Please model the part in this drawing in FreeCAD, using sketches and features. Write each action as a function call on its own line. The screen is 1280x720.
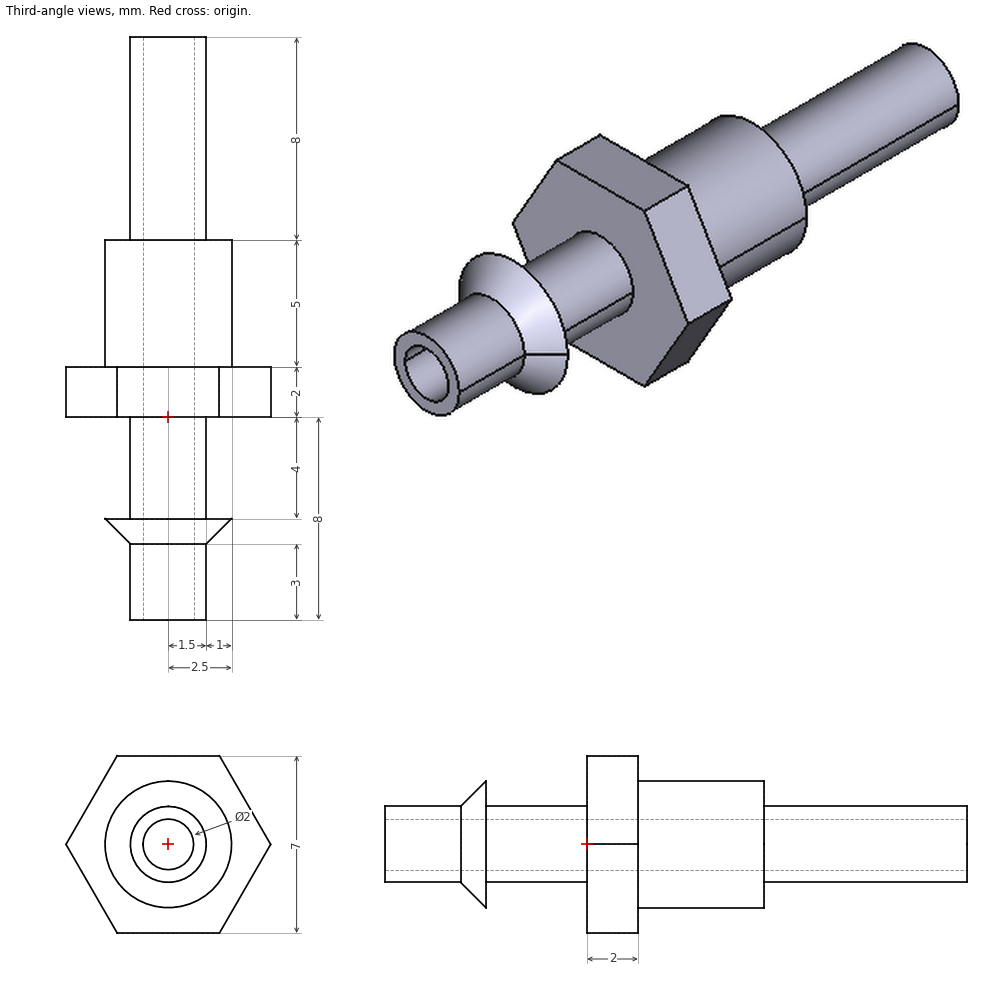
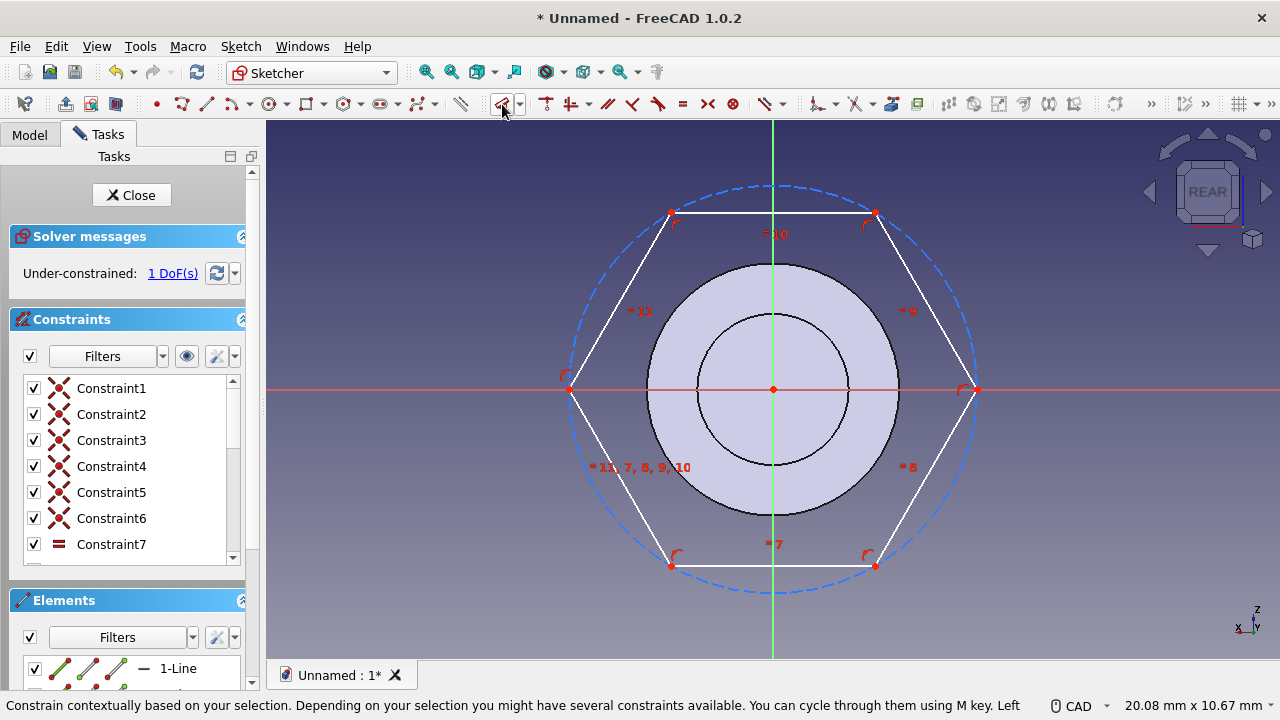
click(671, 566)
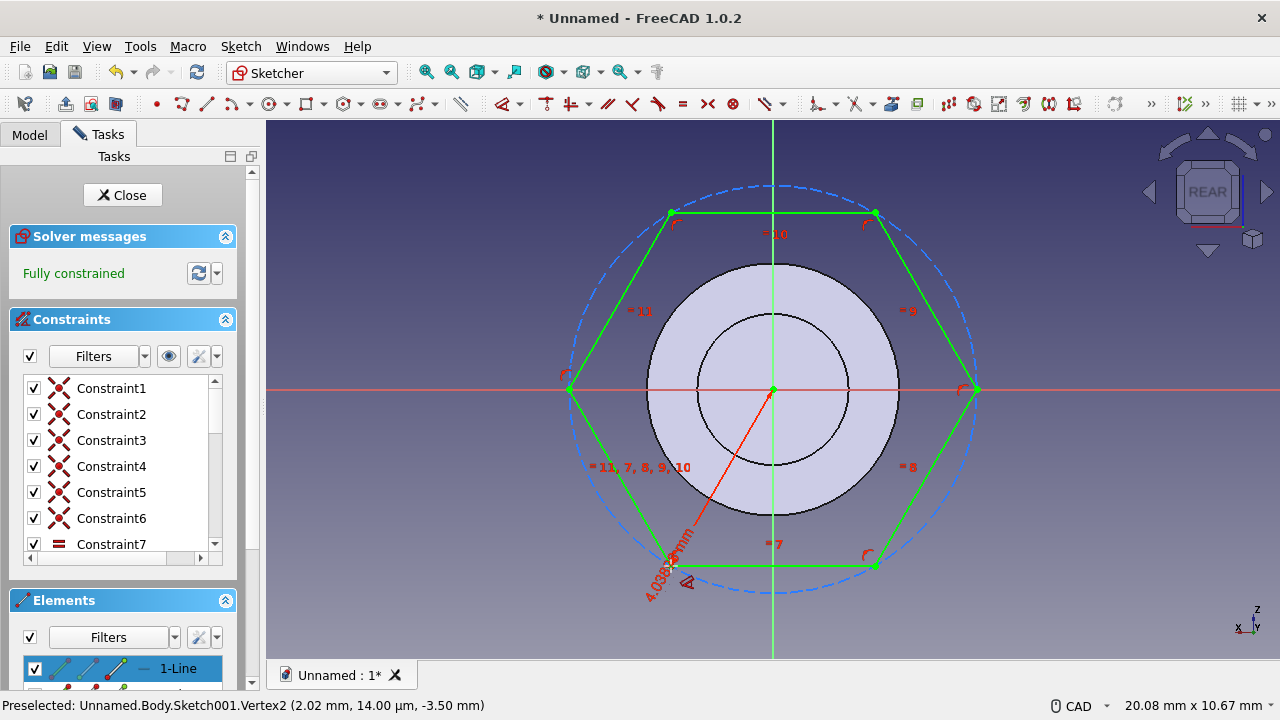
click(875, 213)
click(909, 308)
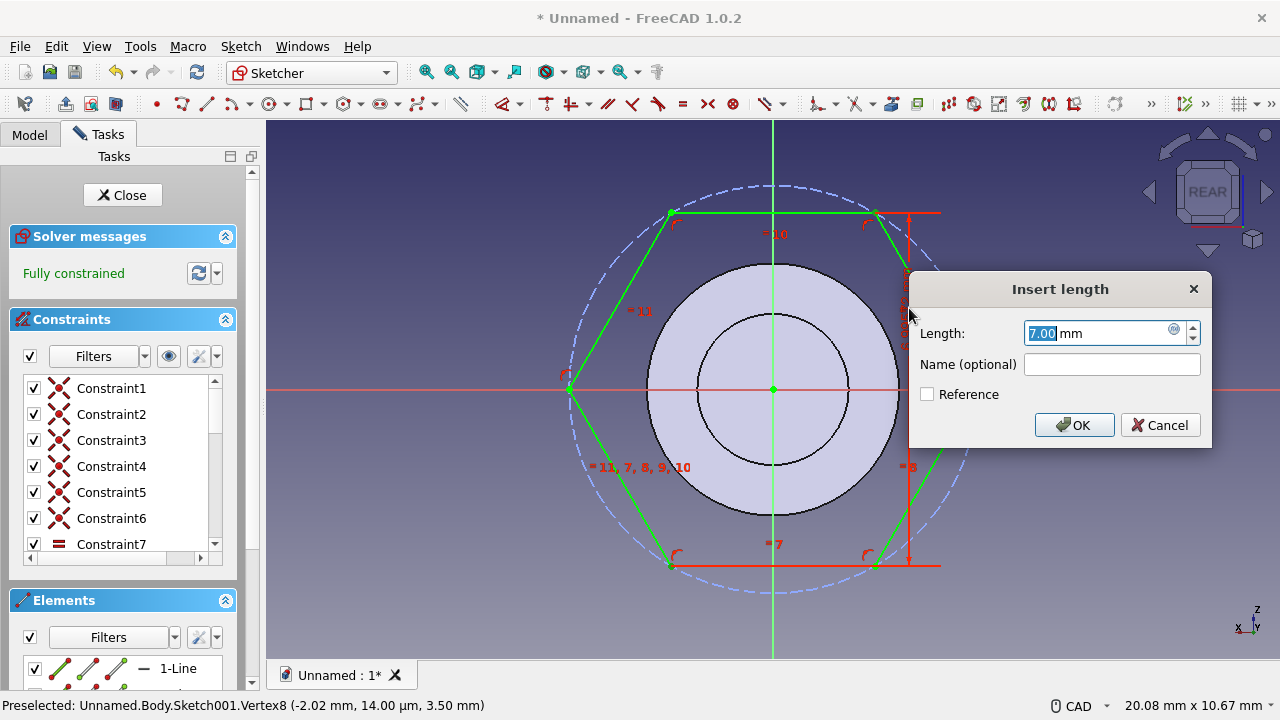
text(7)
key(Return)
key(Escape)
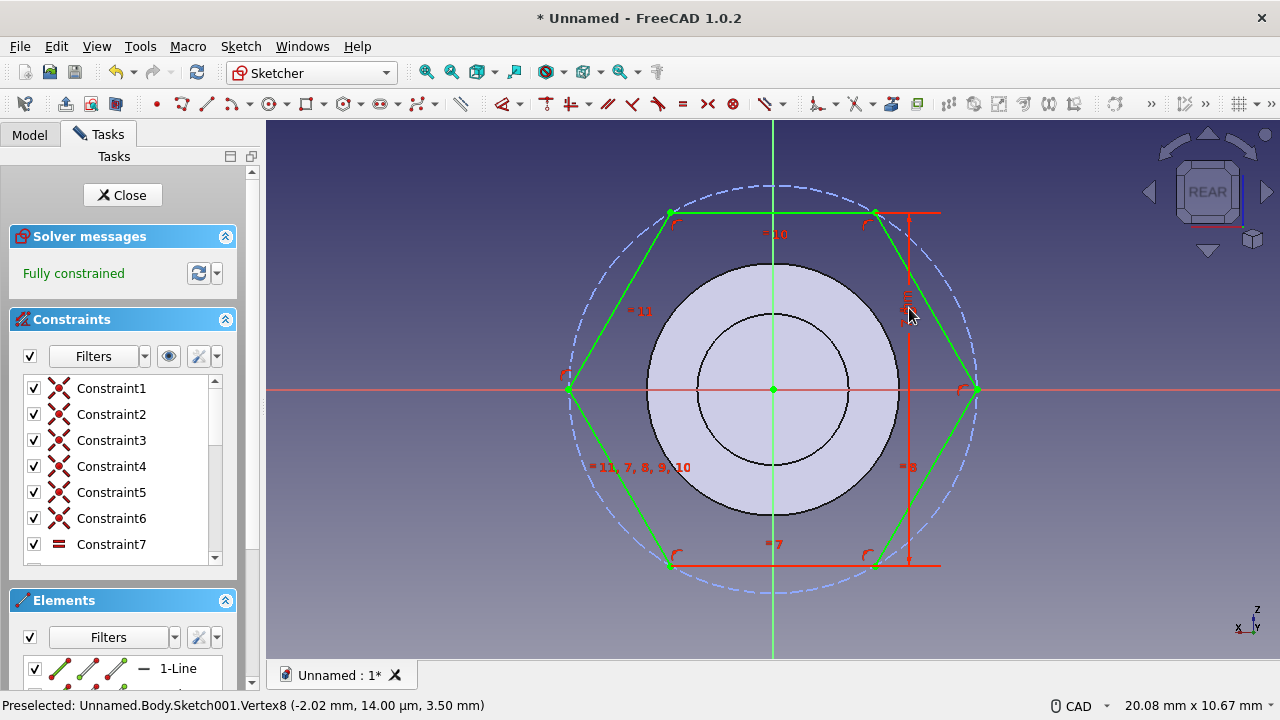
click(123, 195)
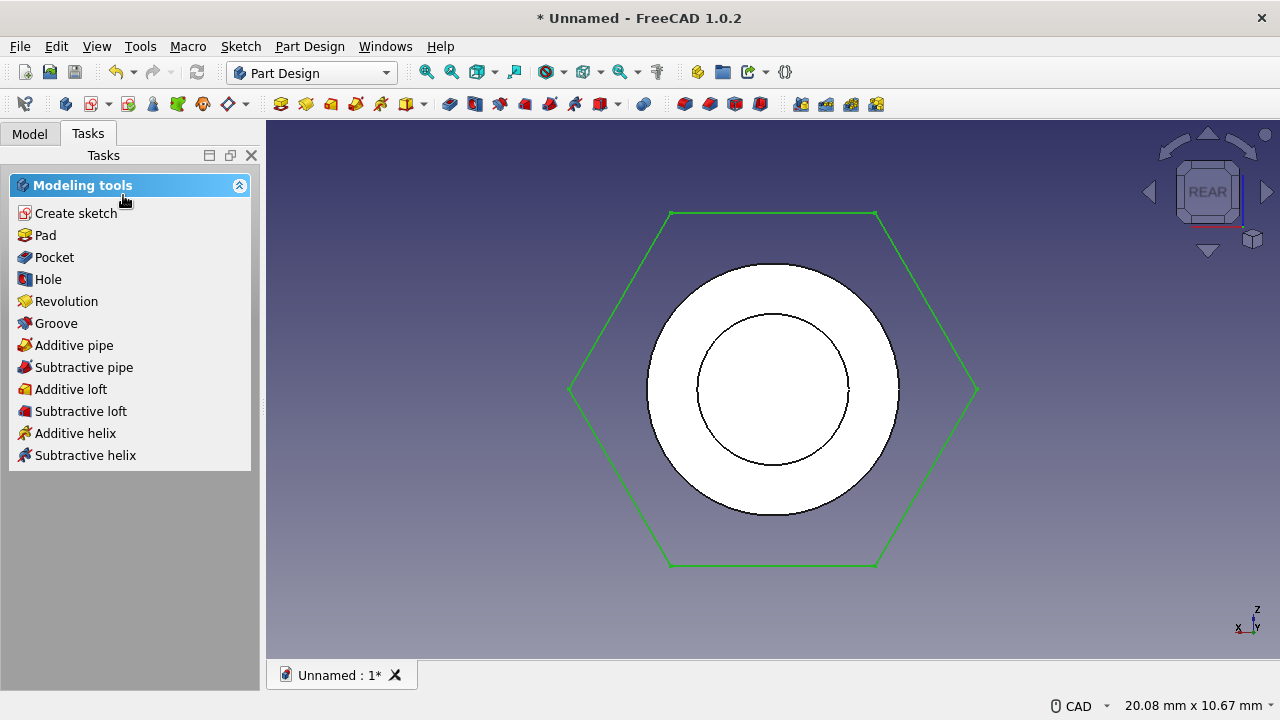
click(281, 104)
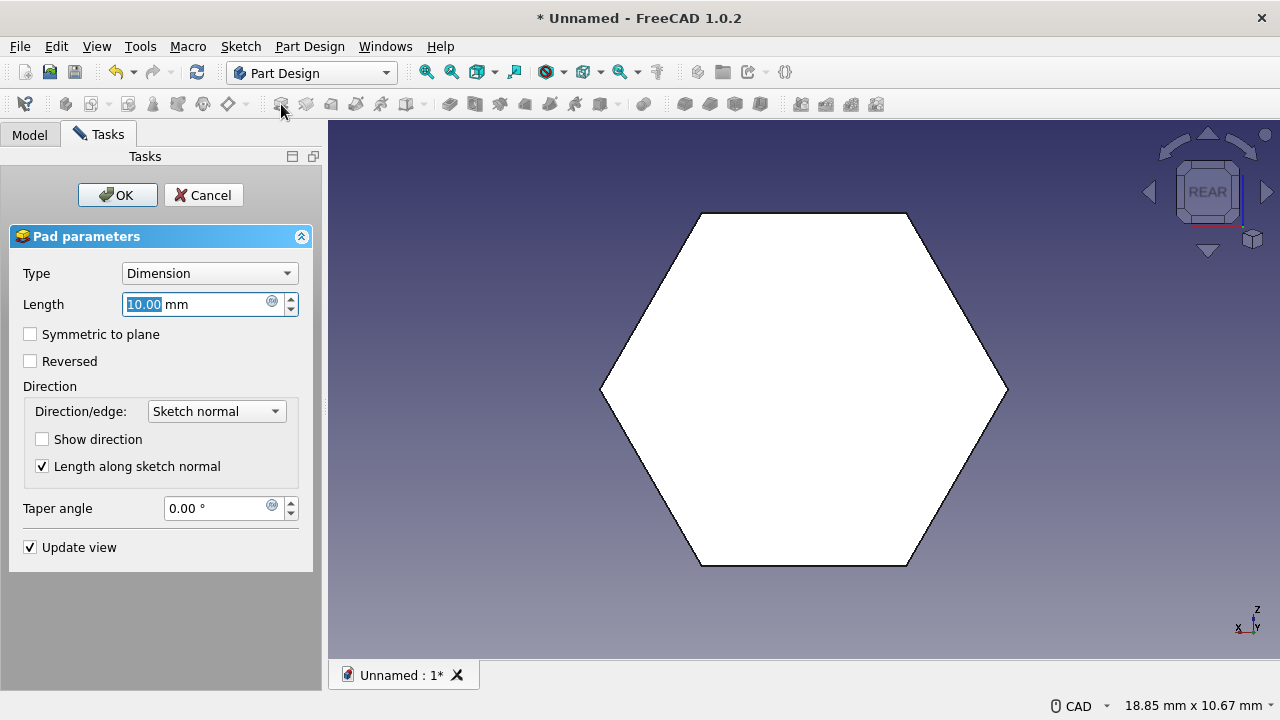
text(2)
key(Tab)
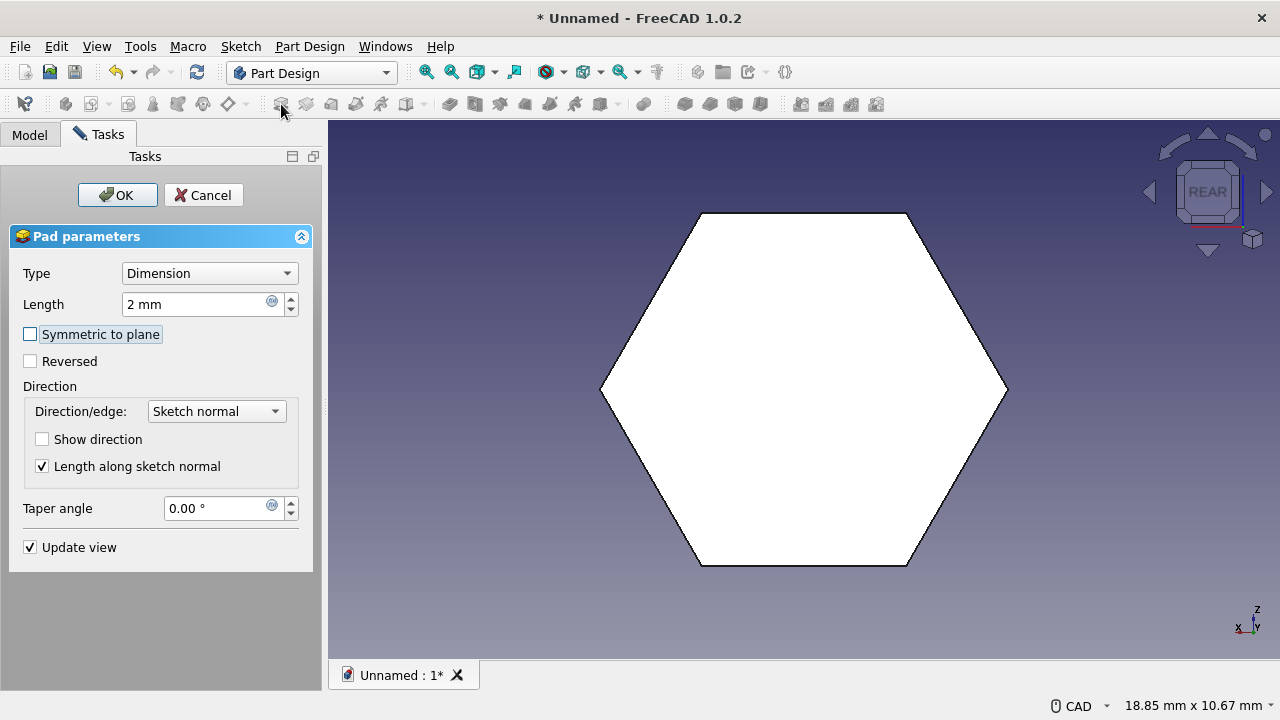
click(118, 195)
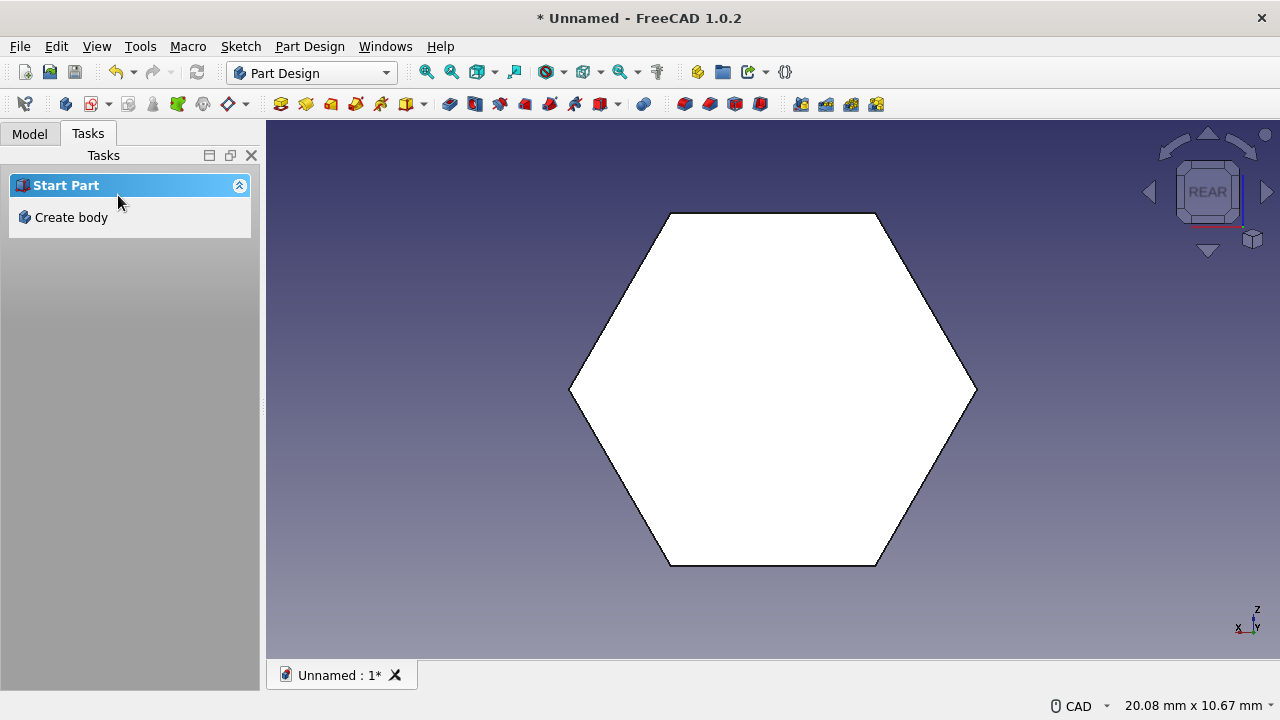
click(90, 104)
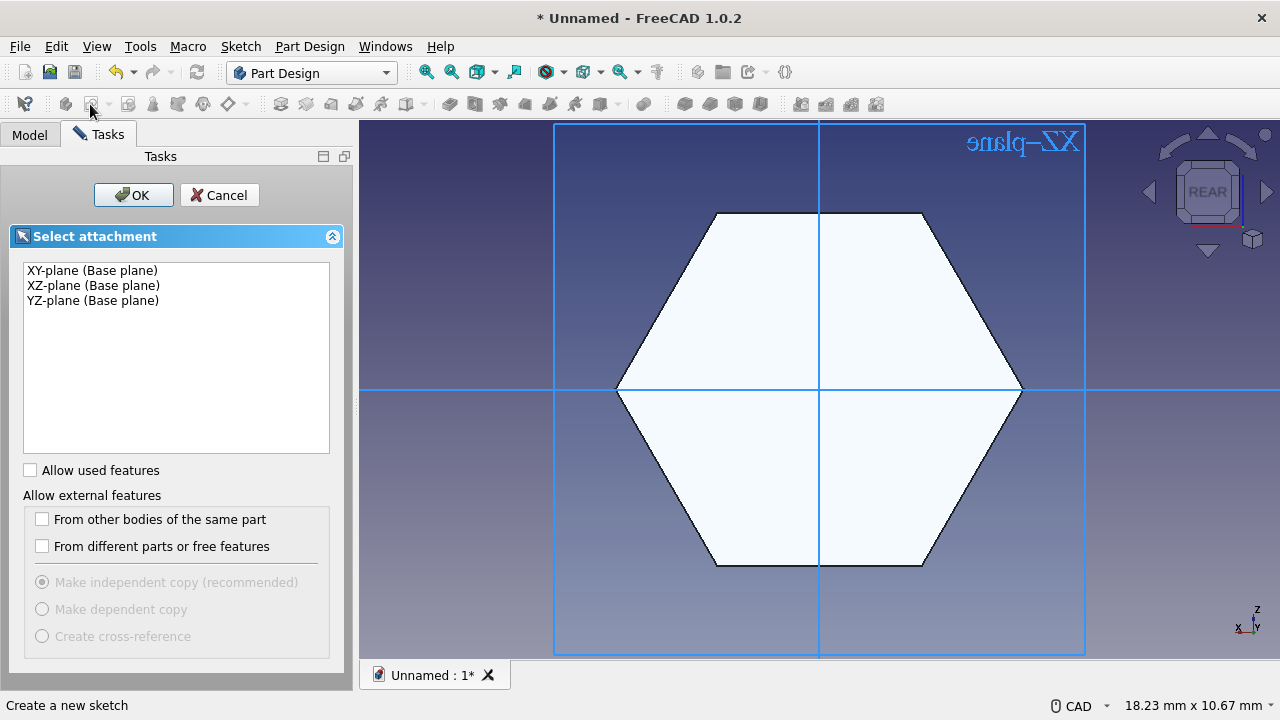
click(84, 270)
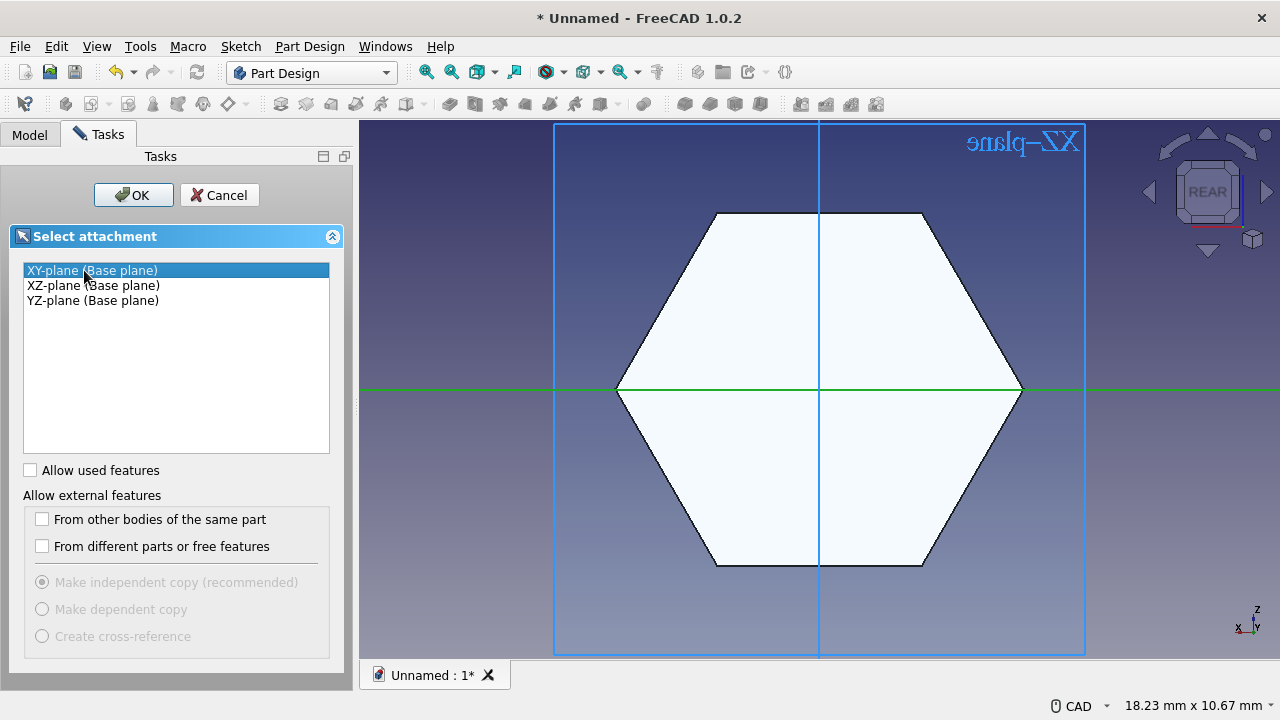
click(134, 195)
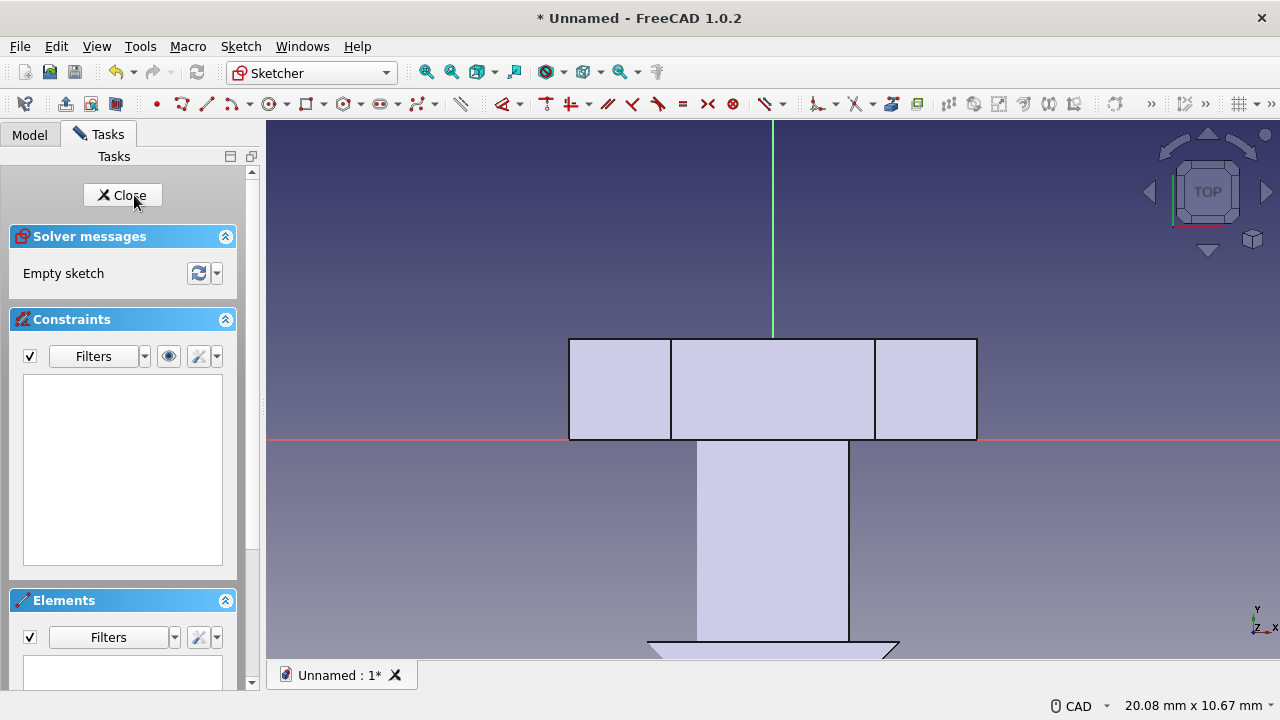
click(116, 104)